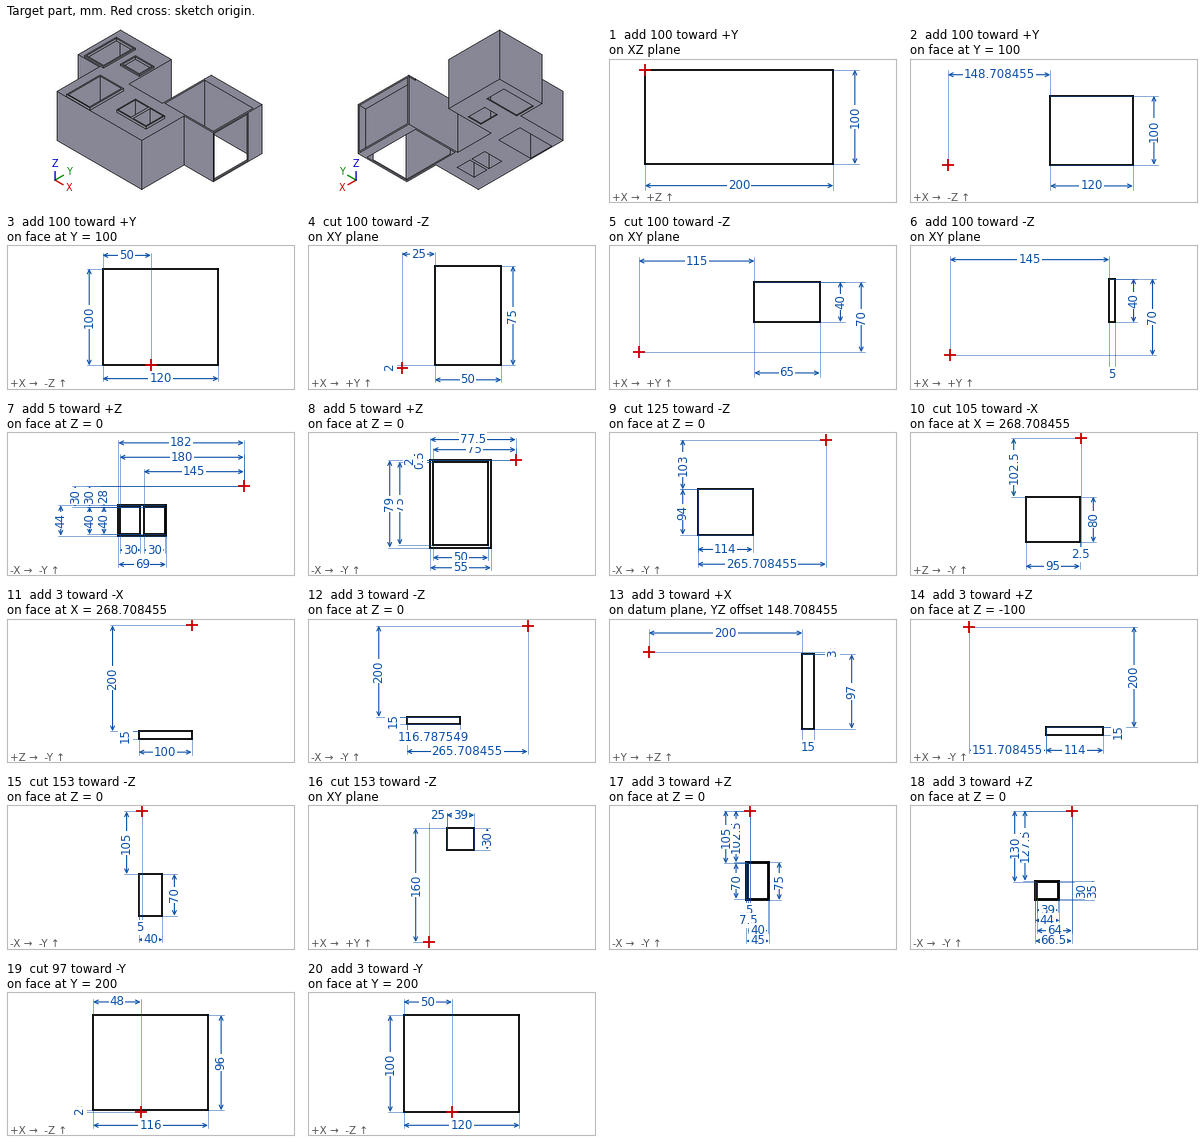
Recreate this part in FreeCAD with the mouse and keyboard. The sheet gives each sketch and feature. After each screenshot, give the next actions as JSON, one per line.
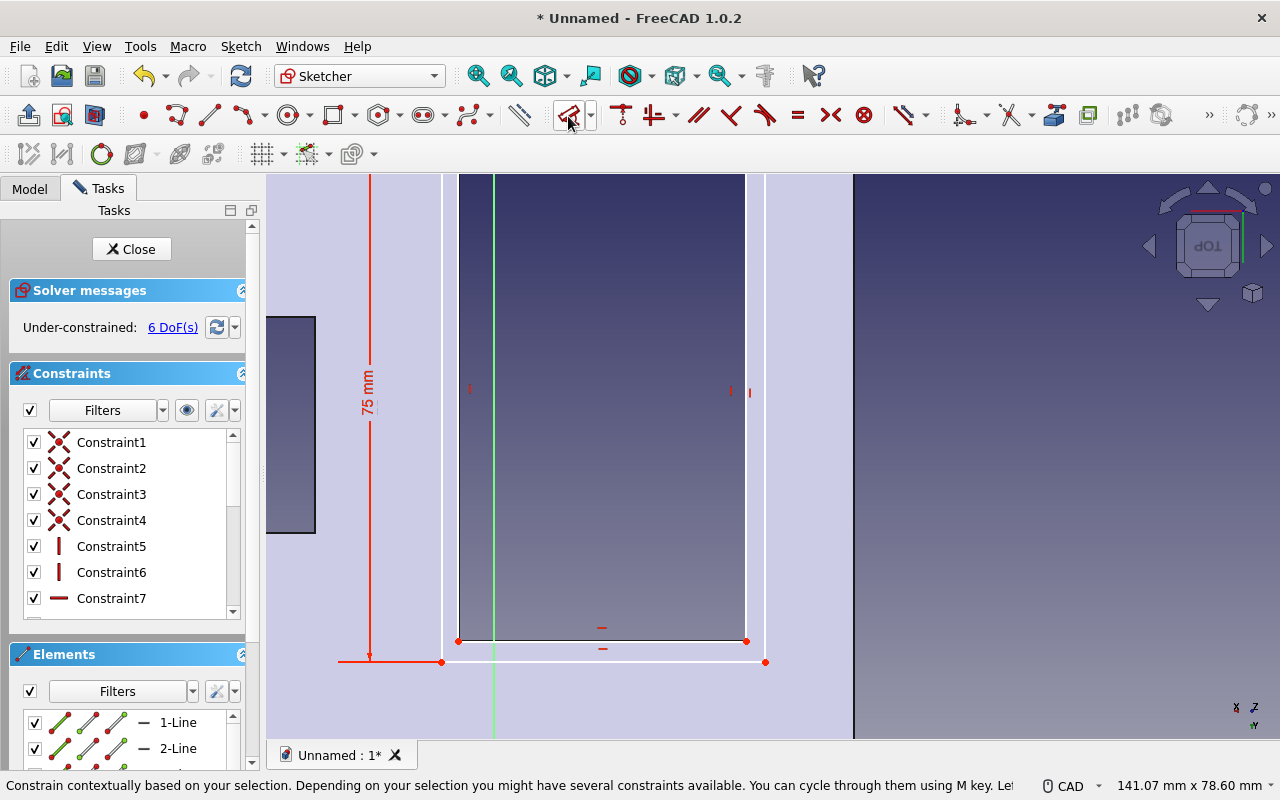
{"action": "left_click", "coordinate": [458, 290]}
{"action": "left_click", "coordinate": [424, 422]}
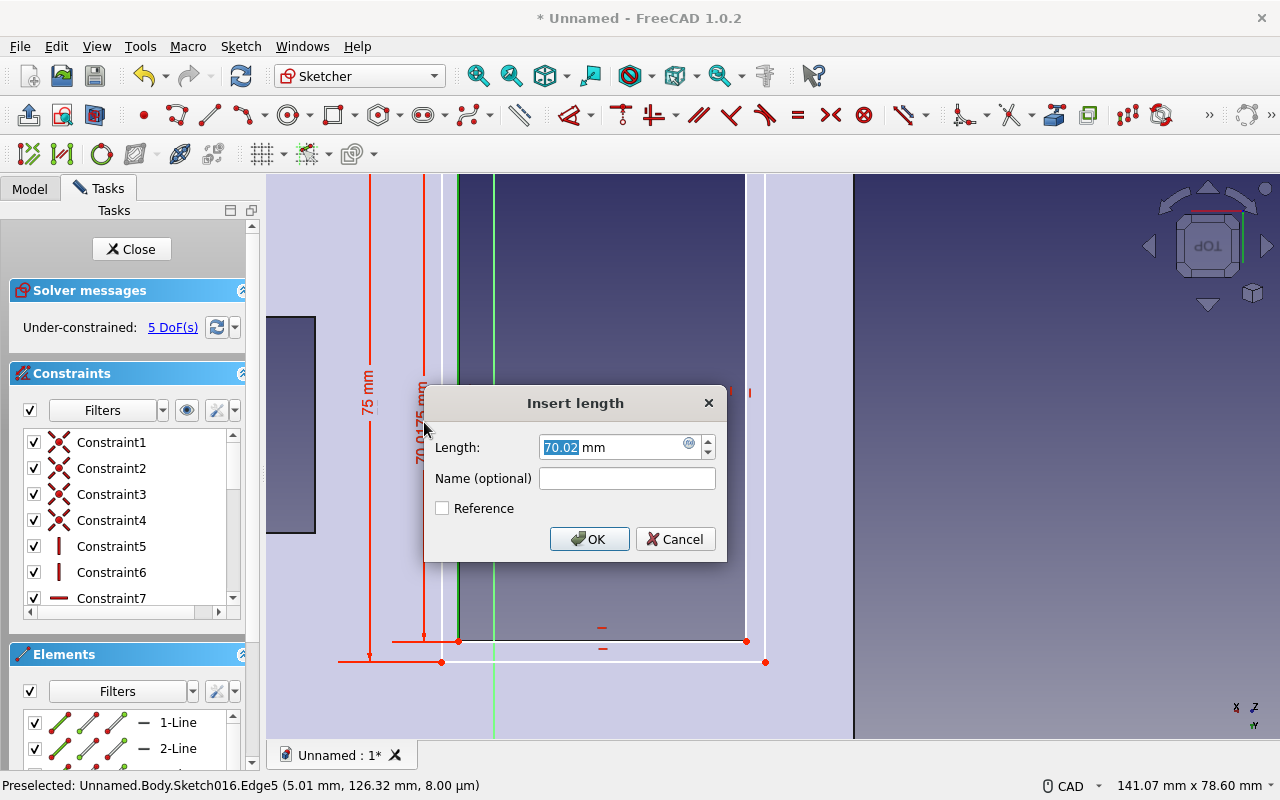
{"action": "type", "text": "70"}
{"action": "key", "text": "Return"}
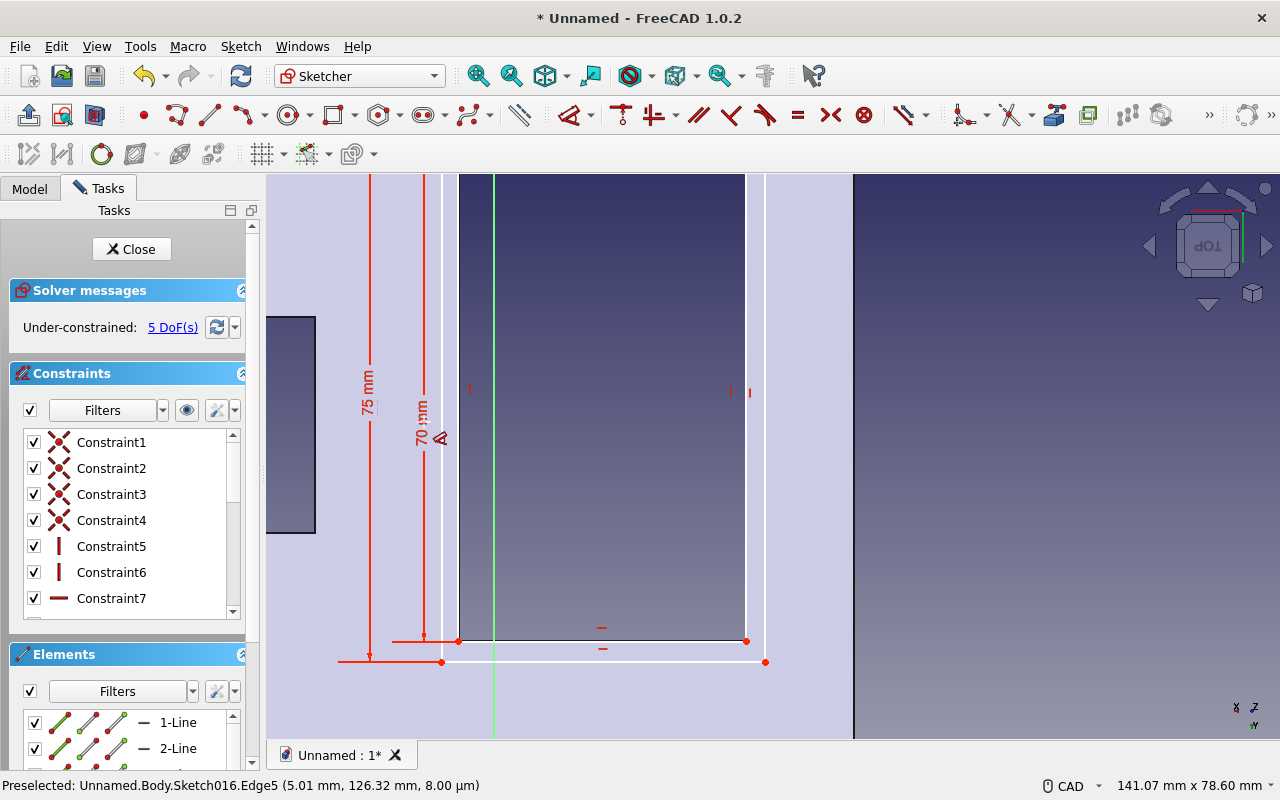
{"action": "left_click", "coordinate": [545, 642]}
{"action": "left_click", "coordinate": [602, 676]}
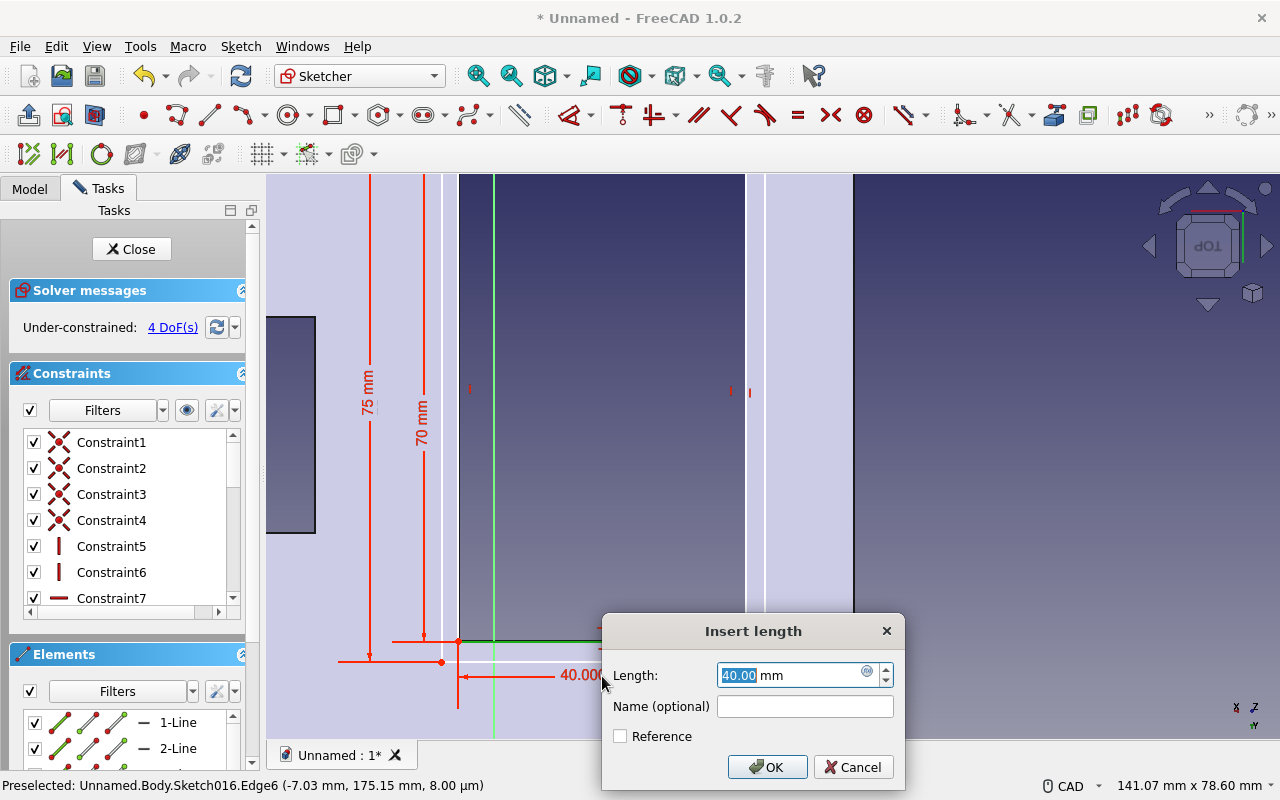
{"action": "type", "text": "40"}
{"action": "key", "text": "Return"}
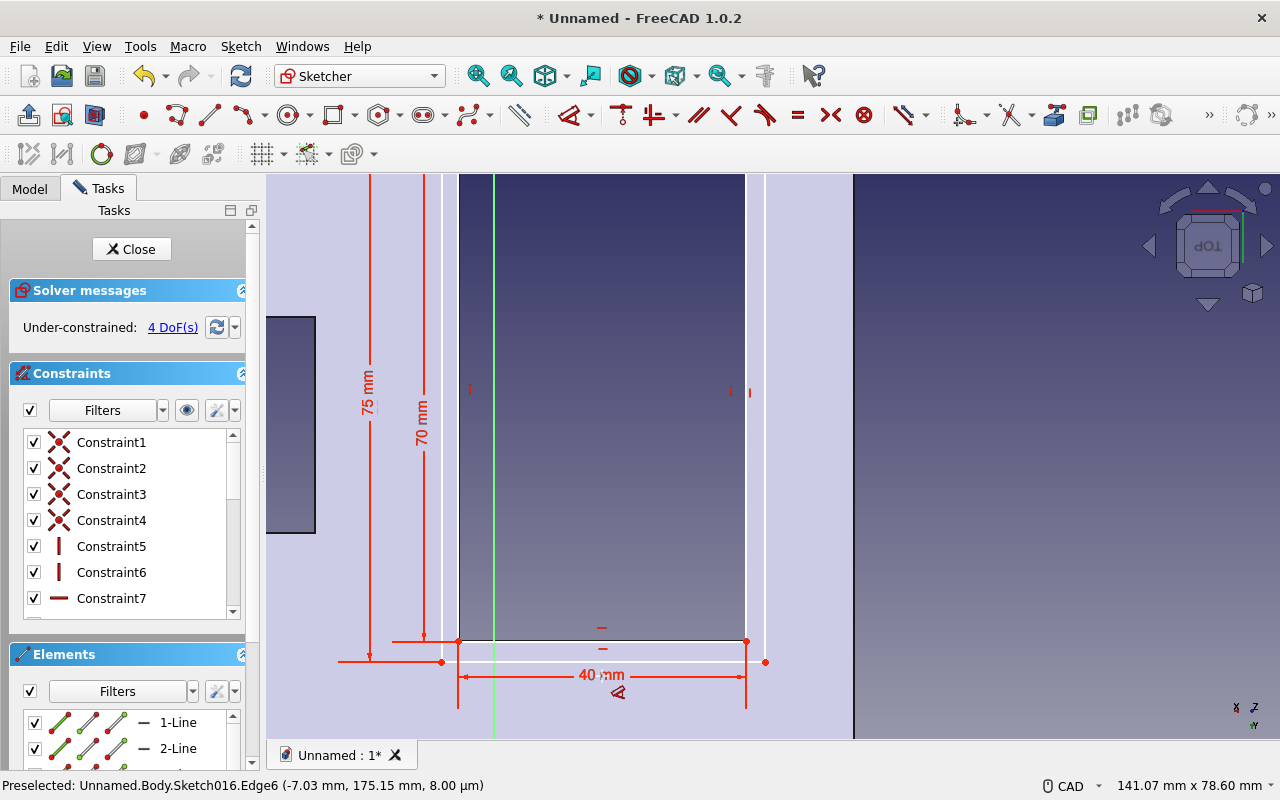
{"action": "scroll", "coordinate": [749, 644], "scroll_direction": "down", "scroll_amount": 6}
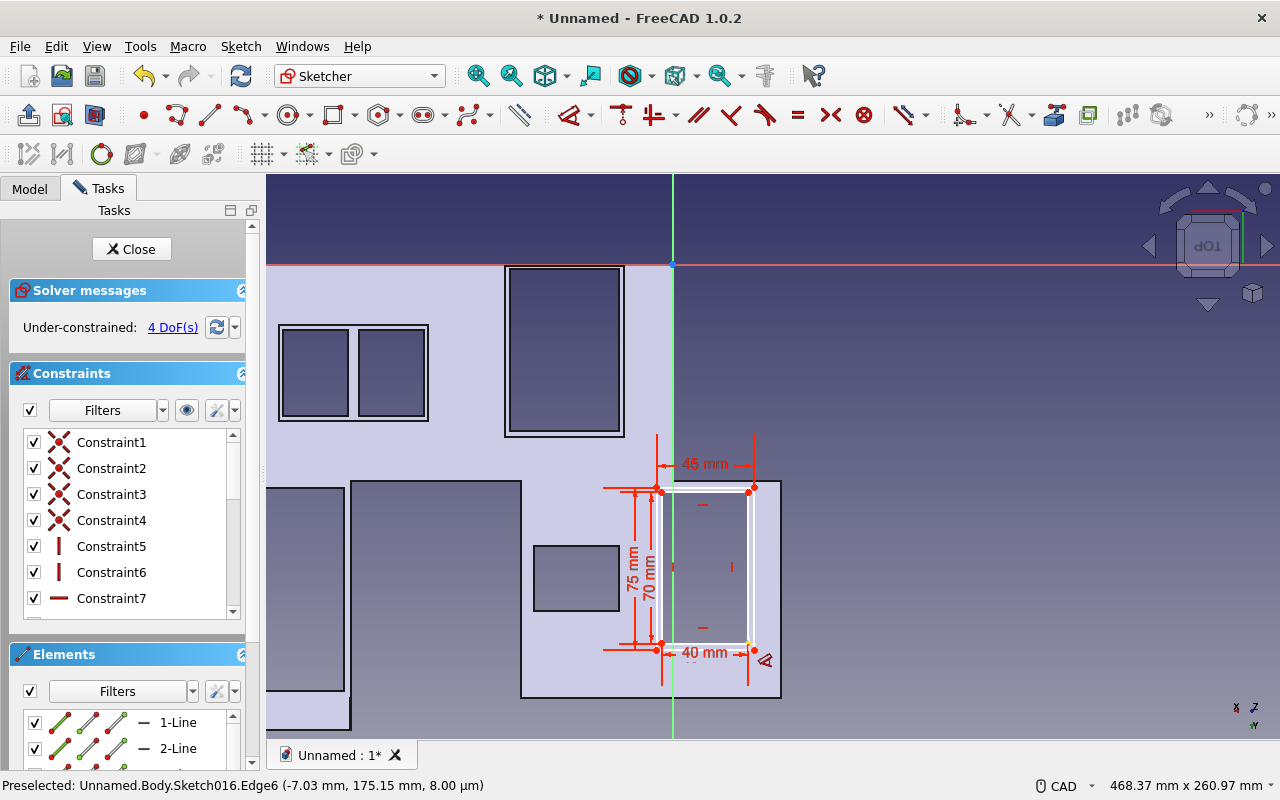
{"action": "scroll", "coordinate": [662, 492], "scroll_direction": "up", "scroll_amount": 7}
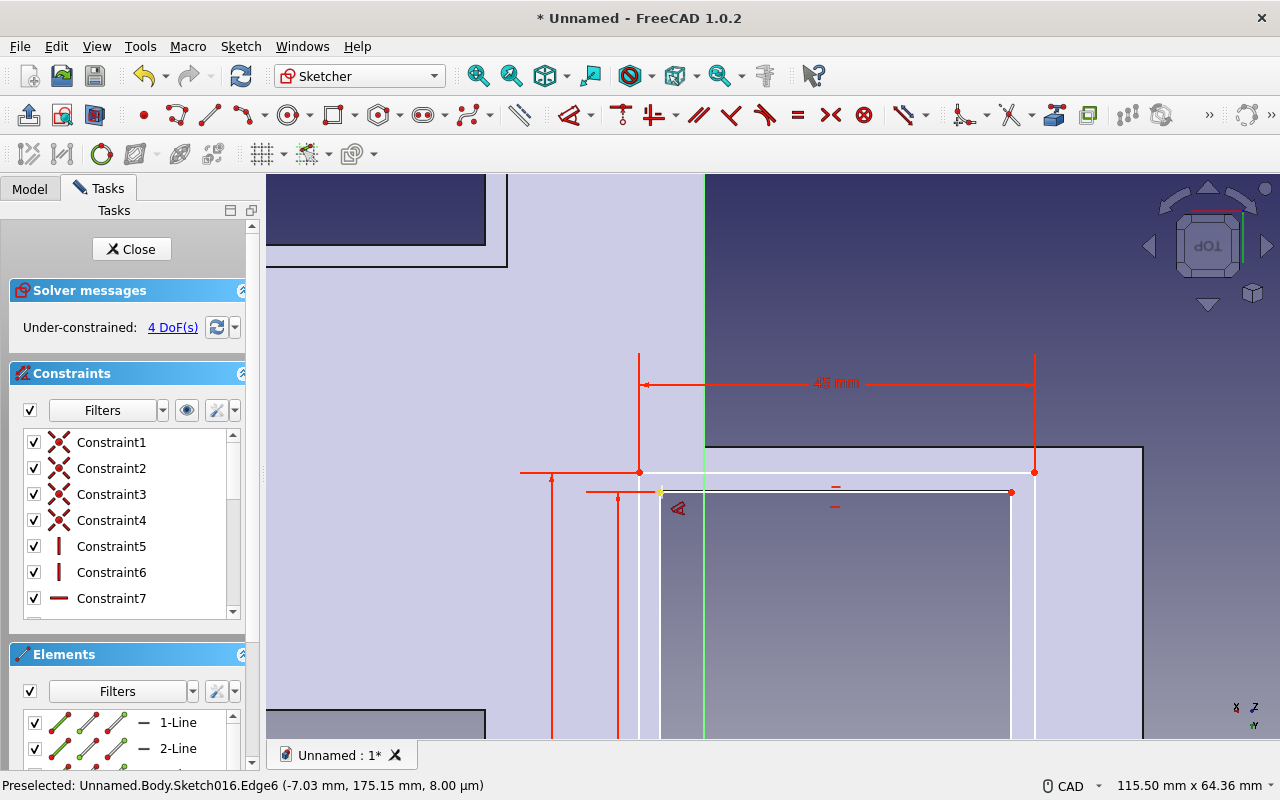
{"action": "left_click", "coordinate": [660, 492]}
{"action": "left_click", "coordinate": [682, 526]}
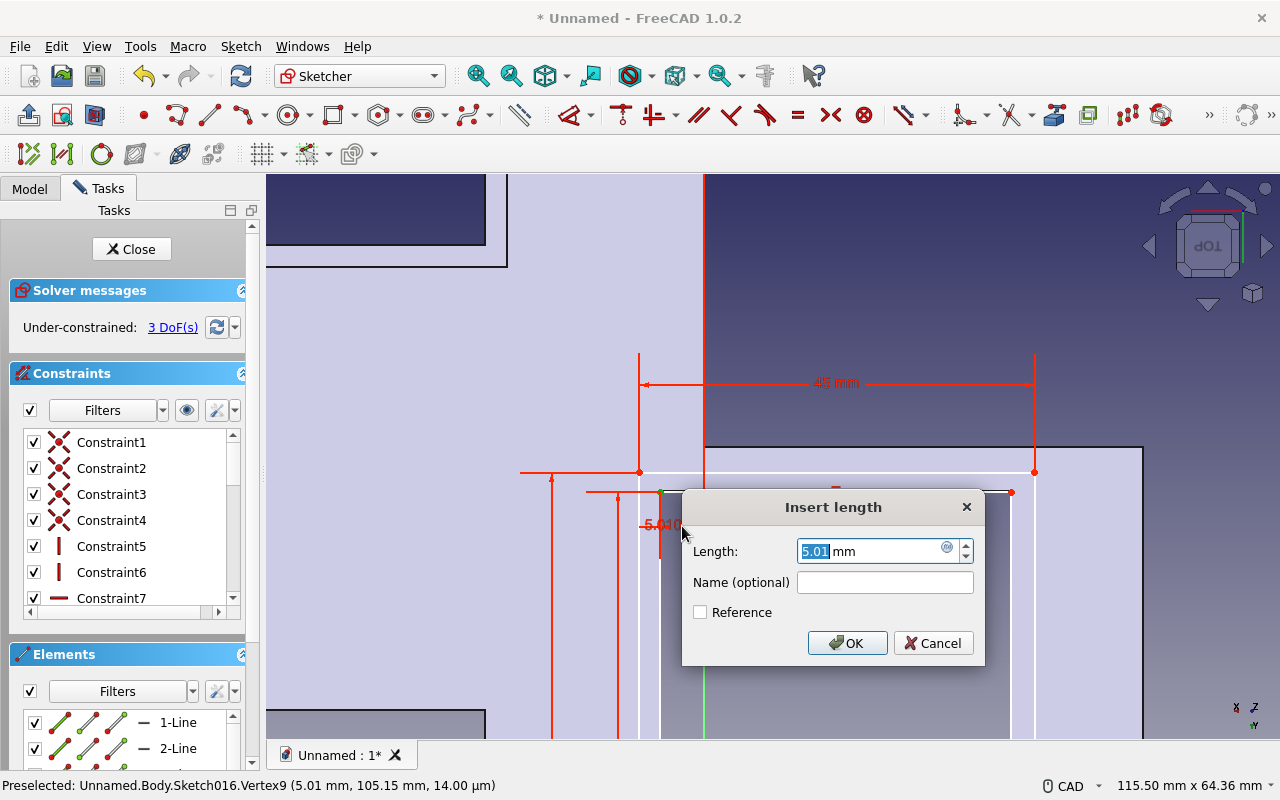
{"action": "type", "text": "5"}
{"action": "key", "text": "Return"}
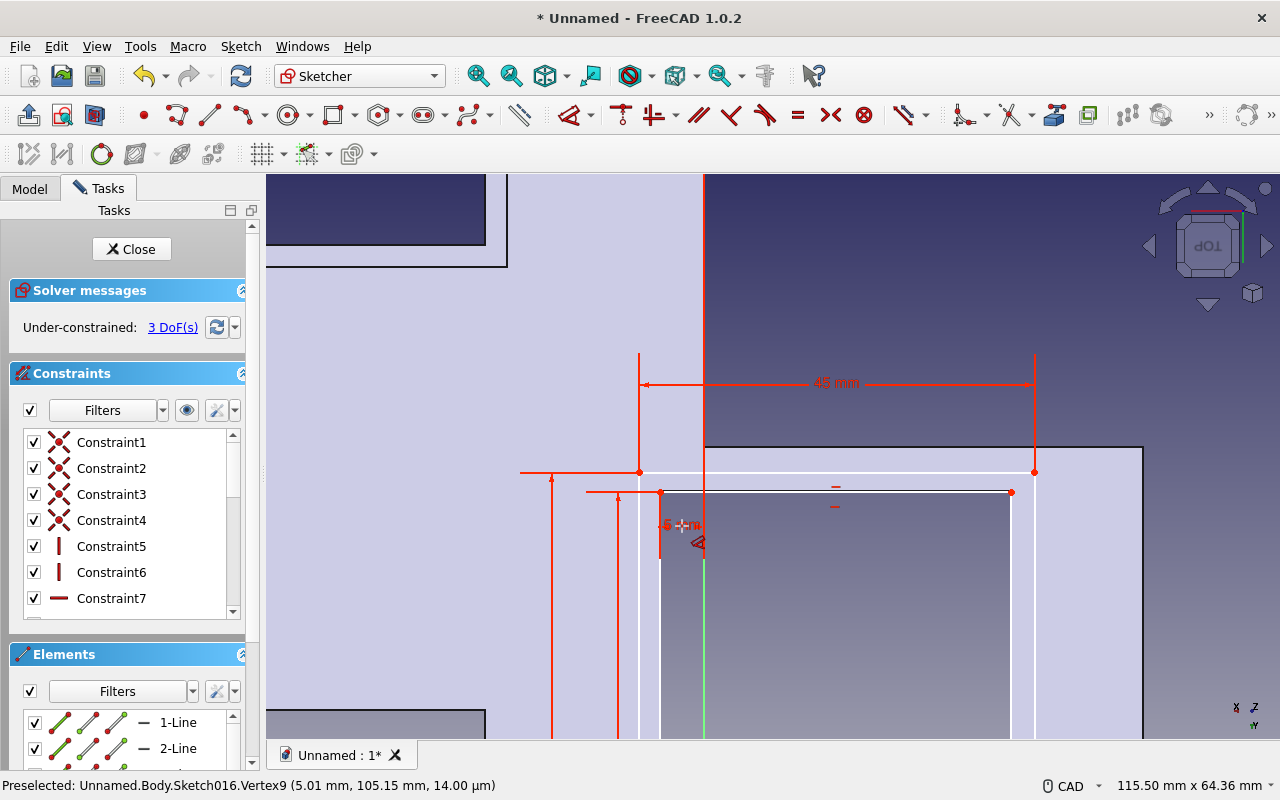
{"action": "left_click", "coordinate": [639, 473]}
{"action": "left_click", "coordinate": [687, 555]}